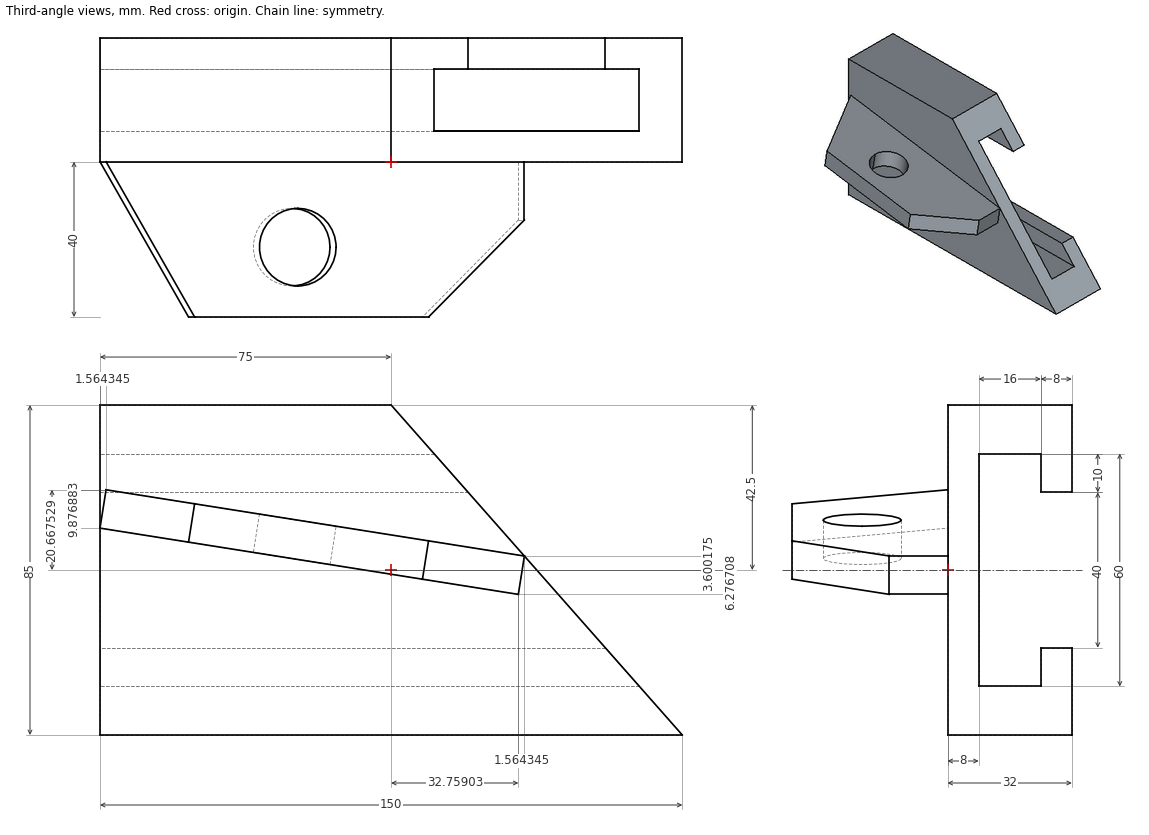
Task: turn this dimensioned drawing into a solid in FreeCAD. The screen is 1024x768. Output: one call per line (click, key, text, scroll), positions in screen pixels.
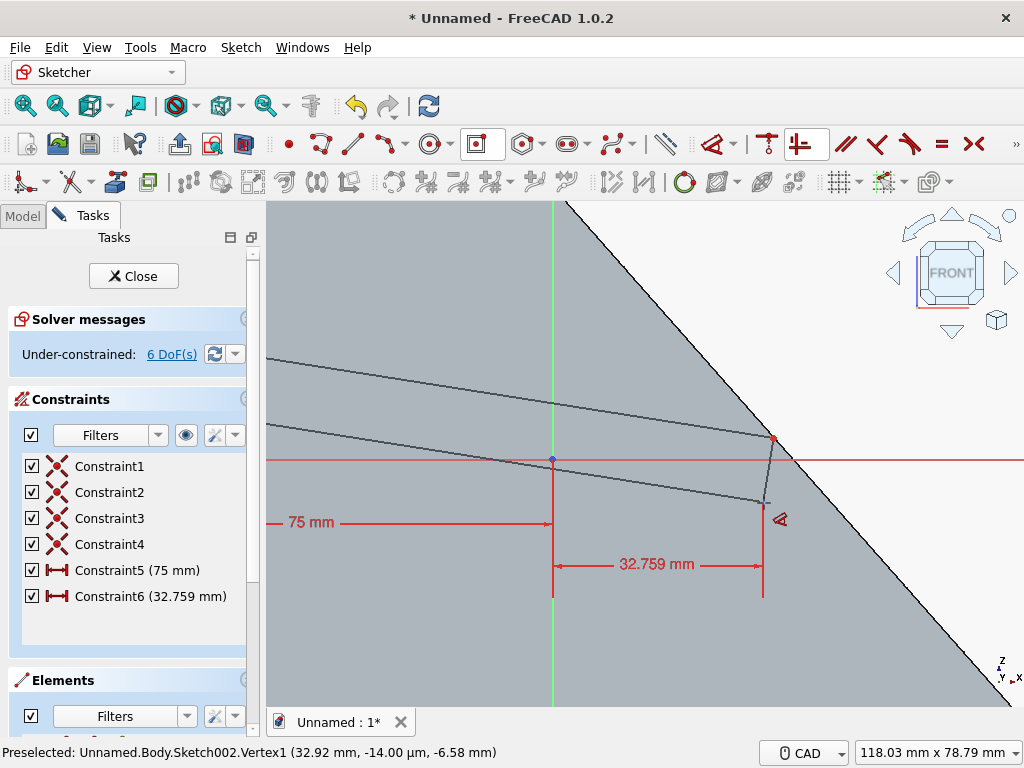
click(763, 502)
click(797, 481)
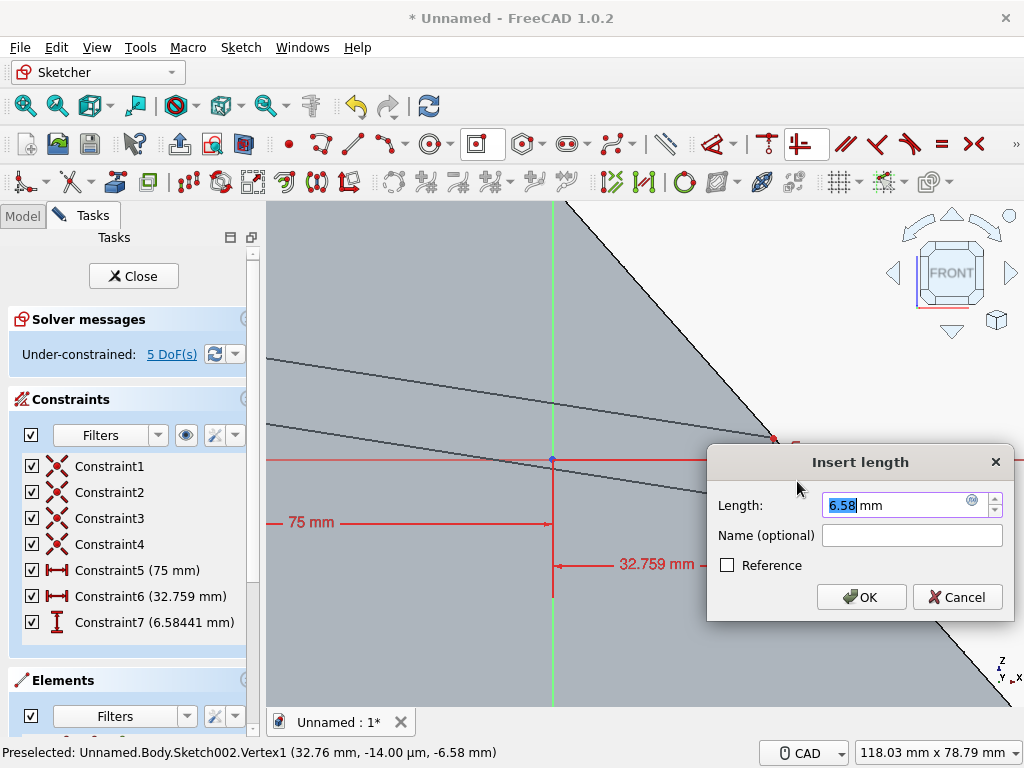
text(6.276708)
key(Return)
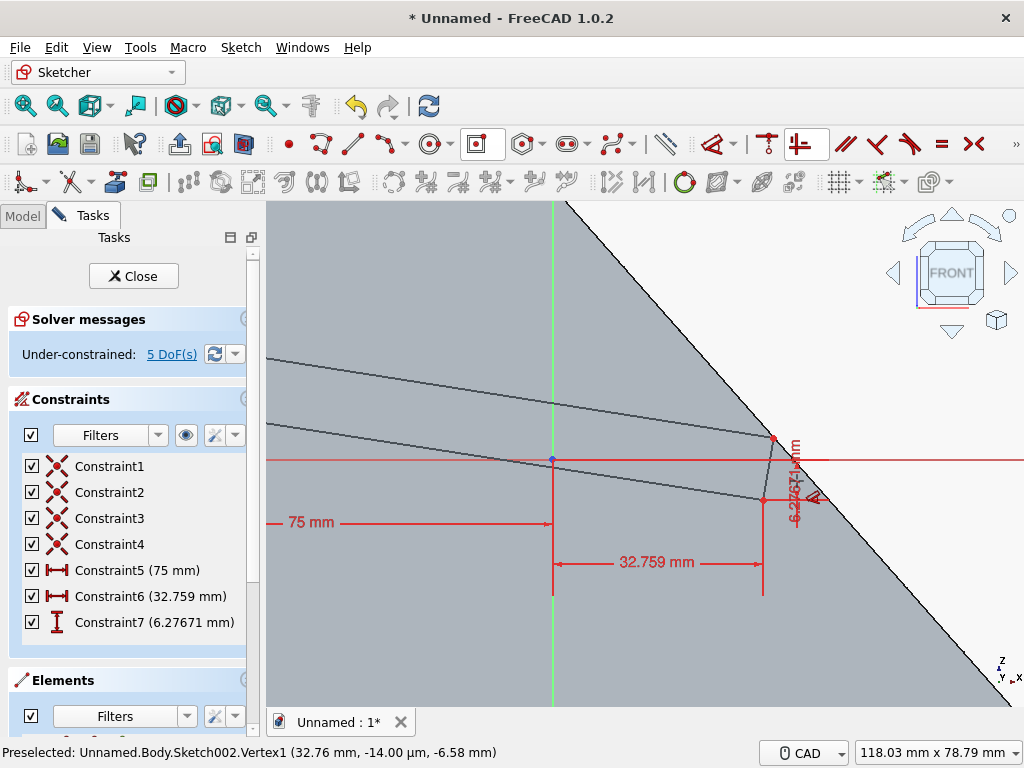
scroll(774, 438, up, 3)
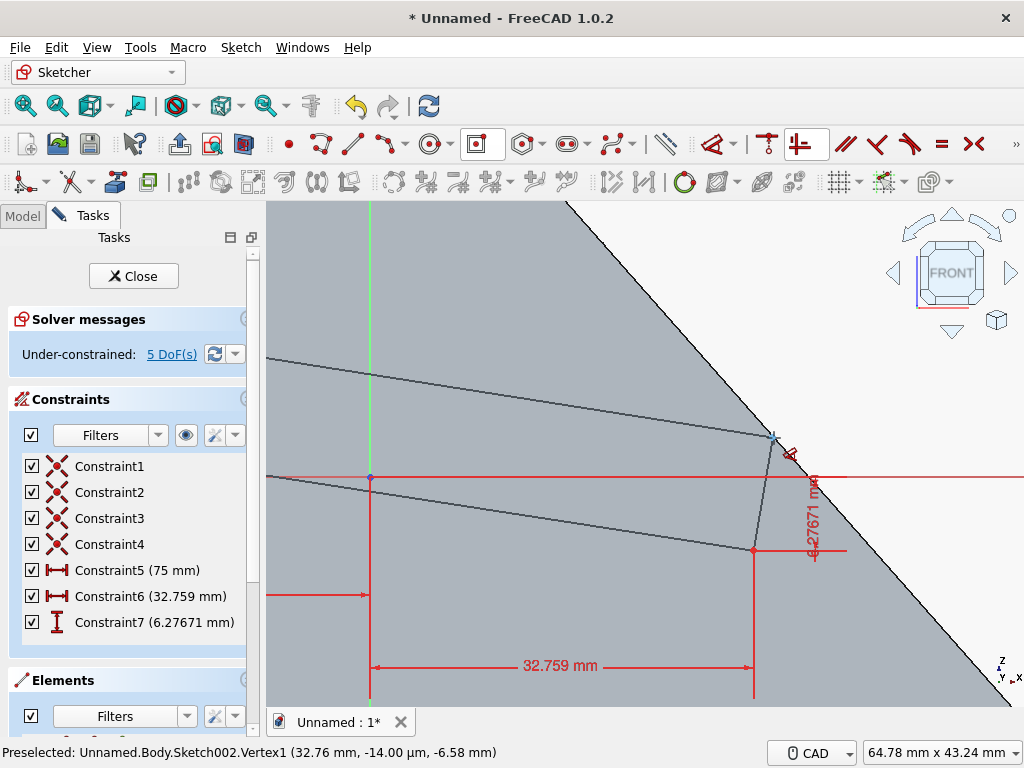
click(773, 438)
click(807, 458)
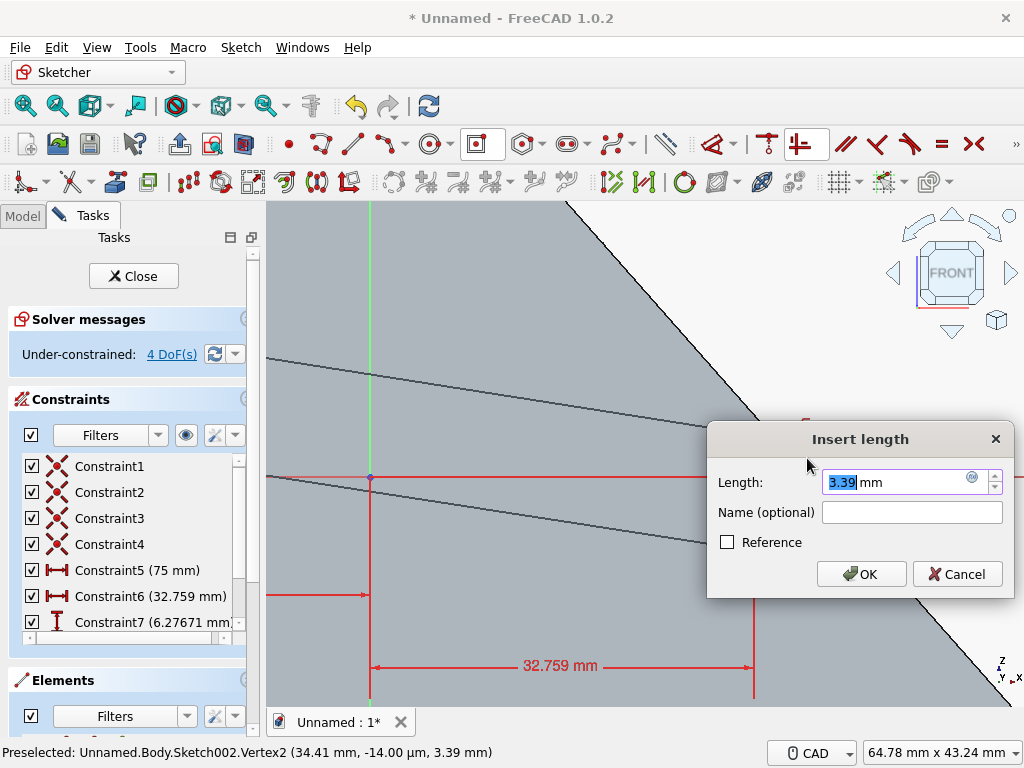
text(3.600175)
key(Return)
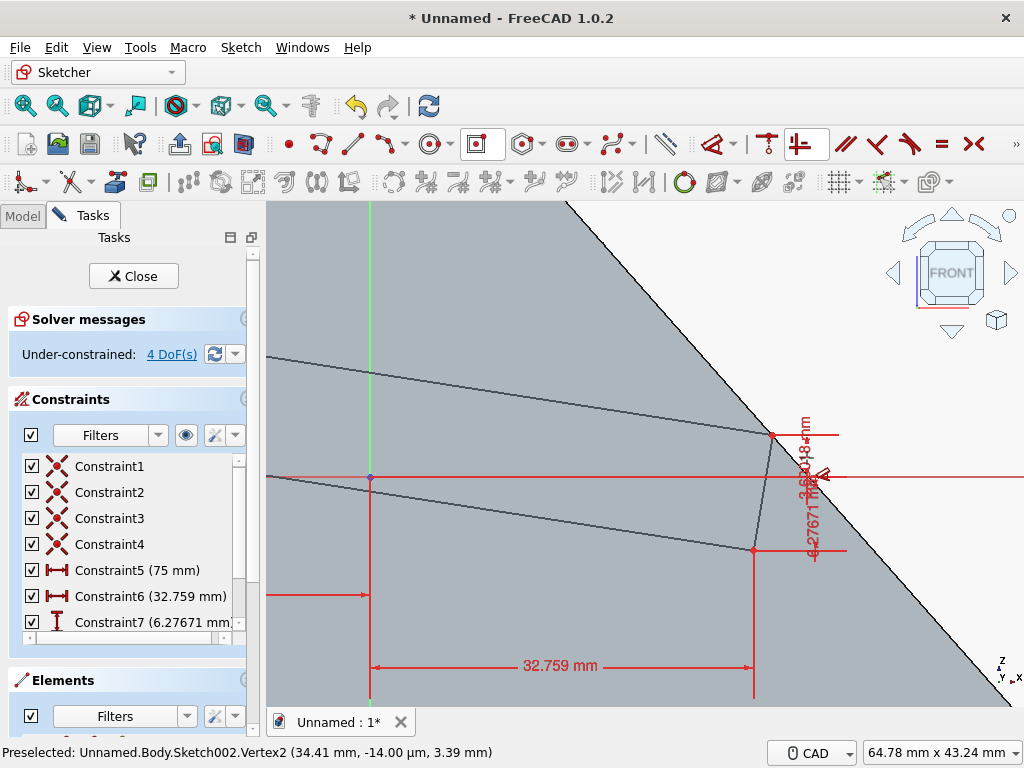
scroll(759, 516, up, 4)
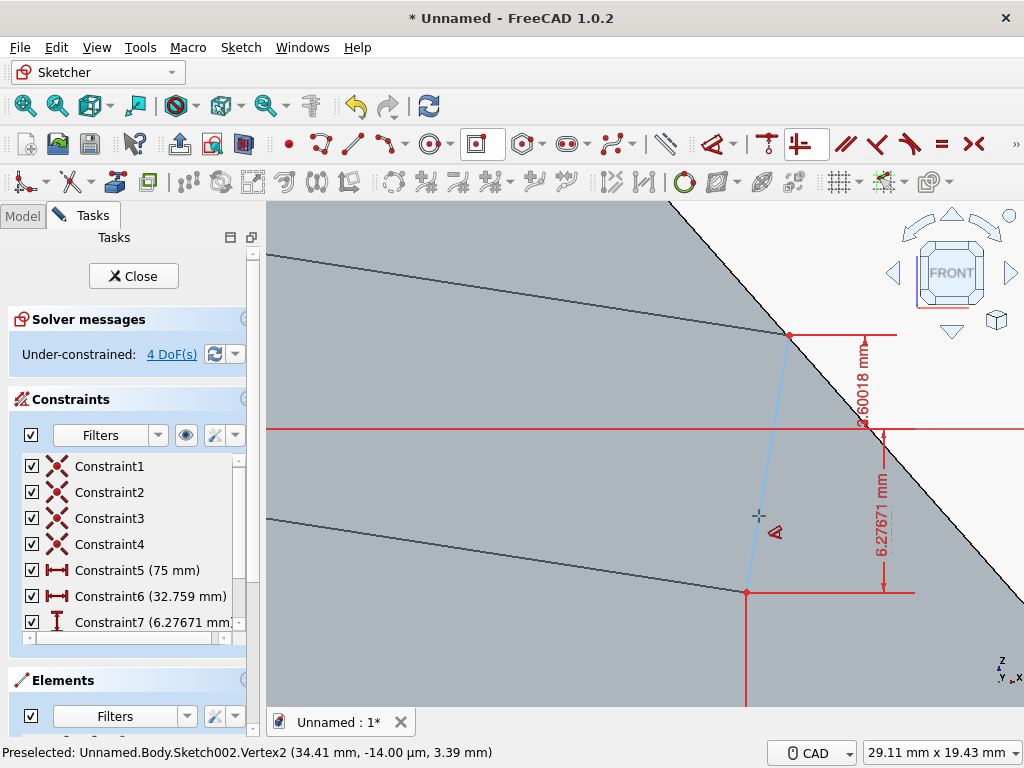
click(759, 515)
click(768, 627)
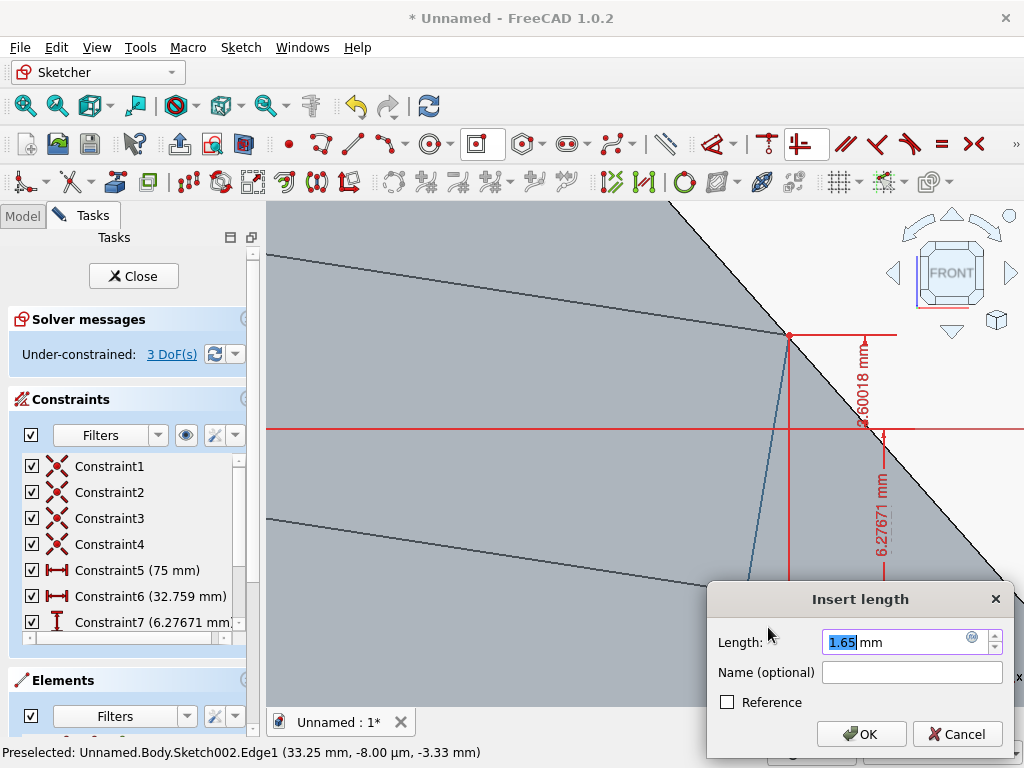
text(1.564345)
key(Return)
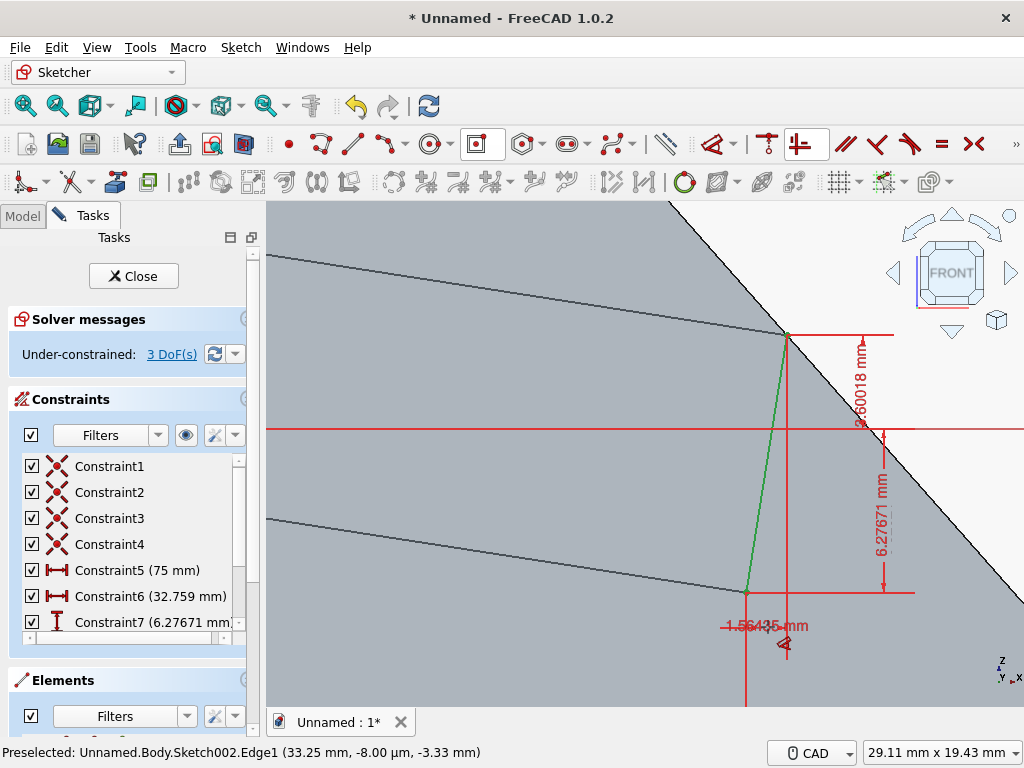
scroll(766, 487, down, 10)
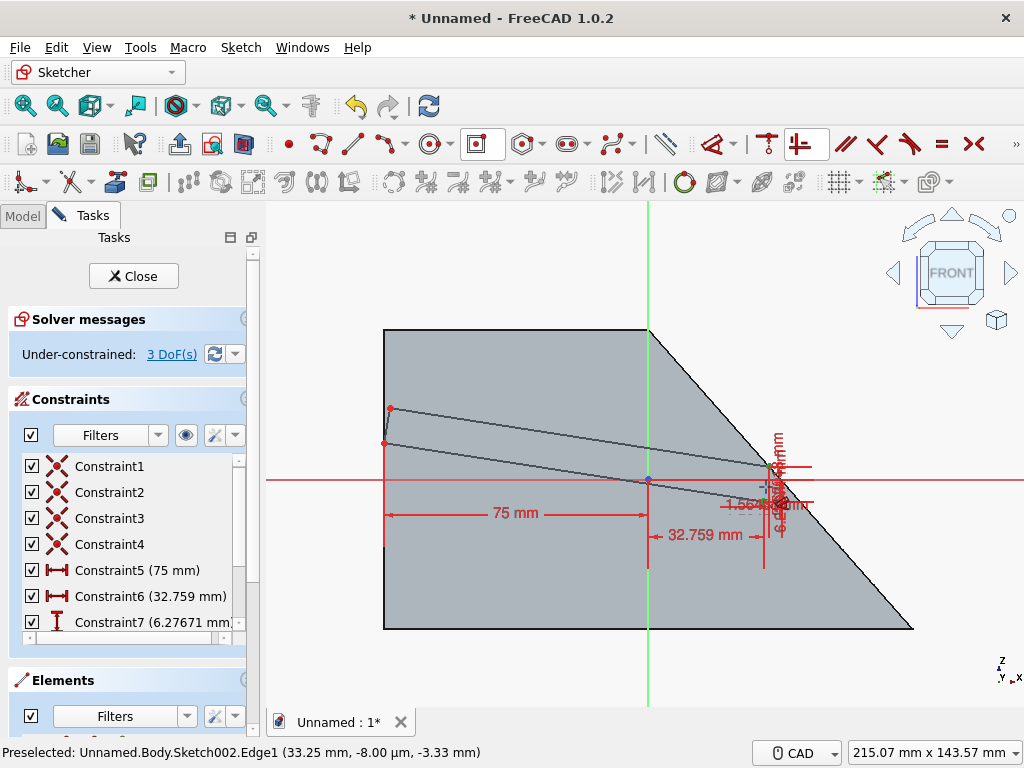
scroll(388, 419, up, 10)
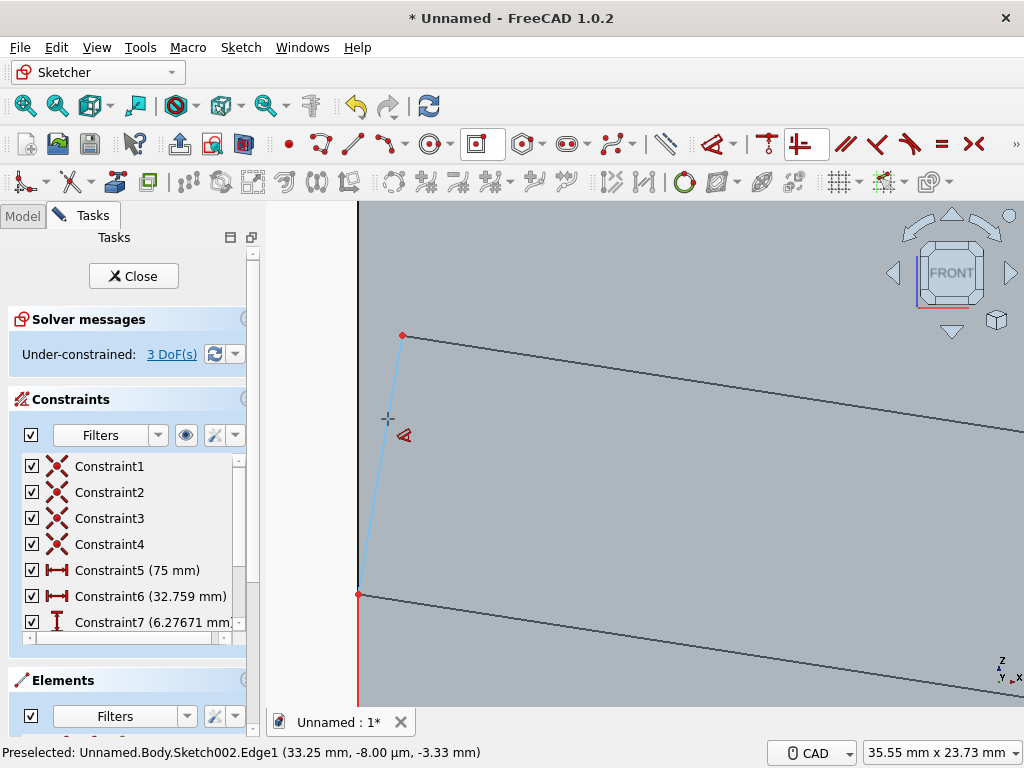
click(389, 413)
click(380, 302)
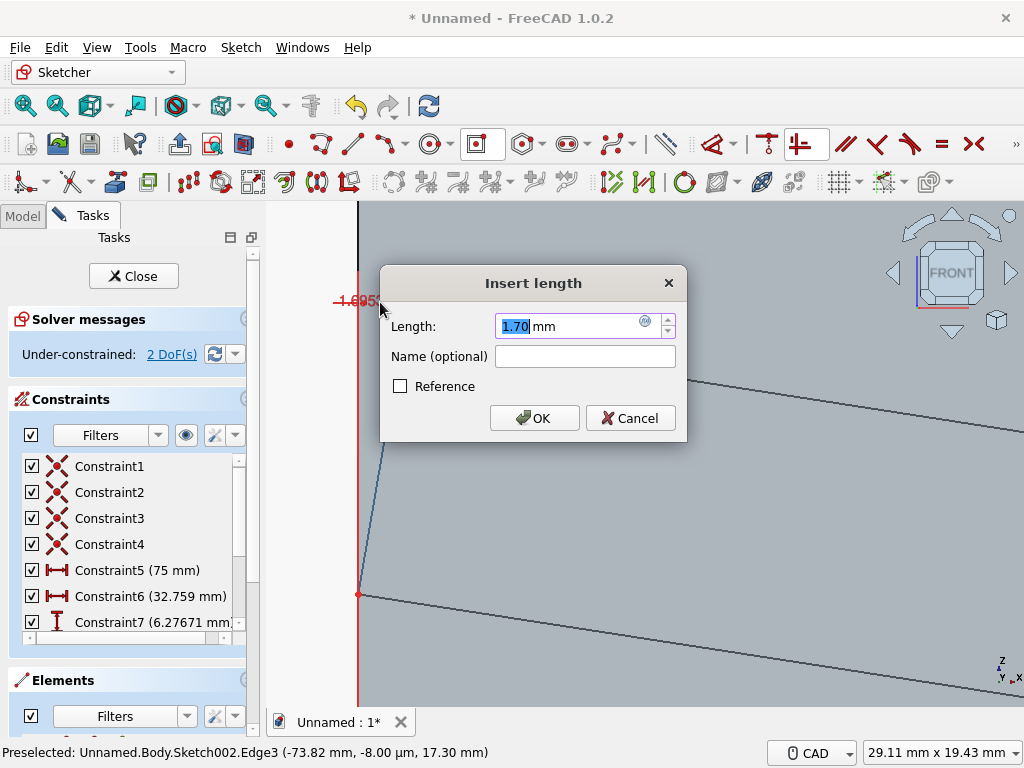
text(1.564345)
key(Return)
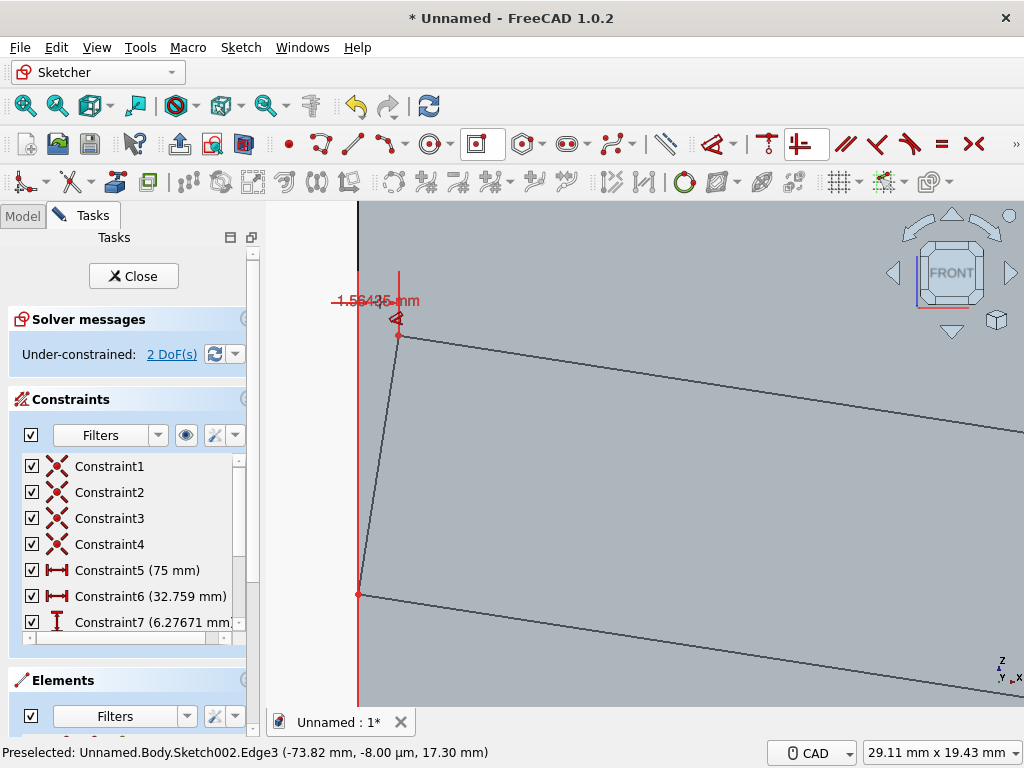
scroll(388, 419, down, 10)